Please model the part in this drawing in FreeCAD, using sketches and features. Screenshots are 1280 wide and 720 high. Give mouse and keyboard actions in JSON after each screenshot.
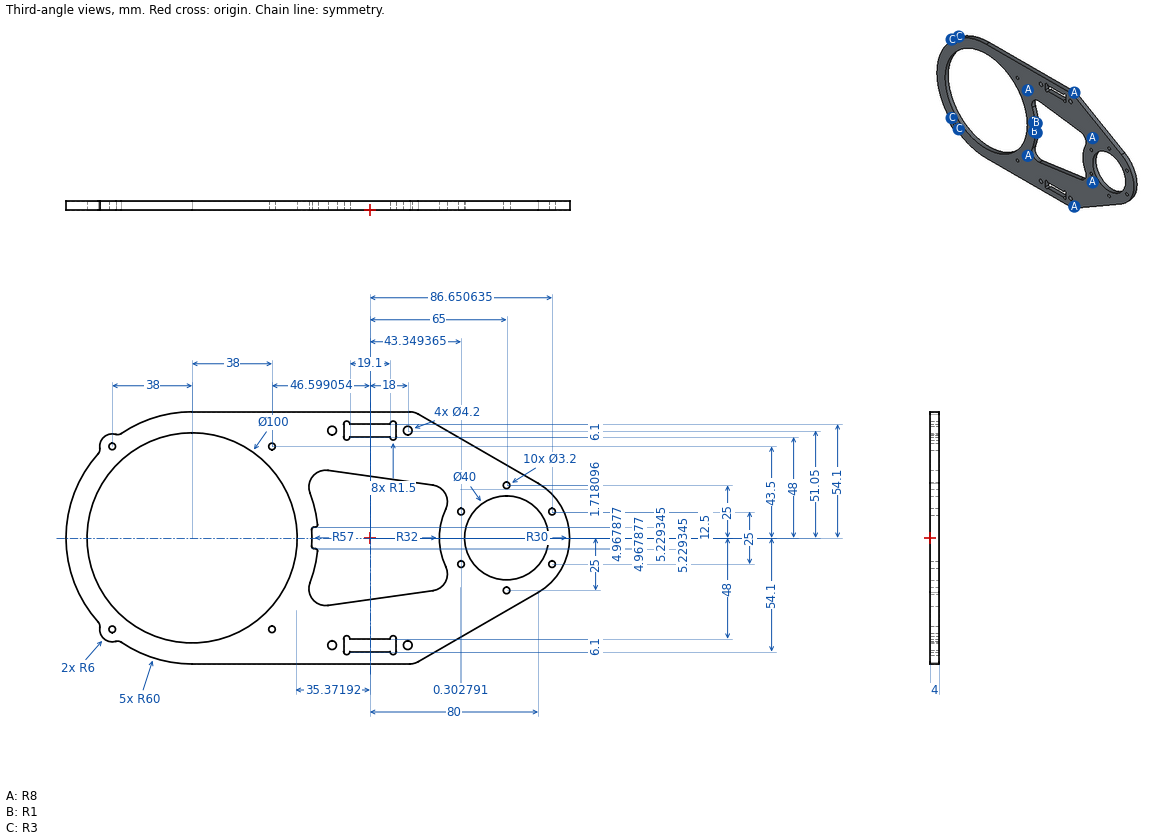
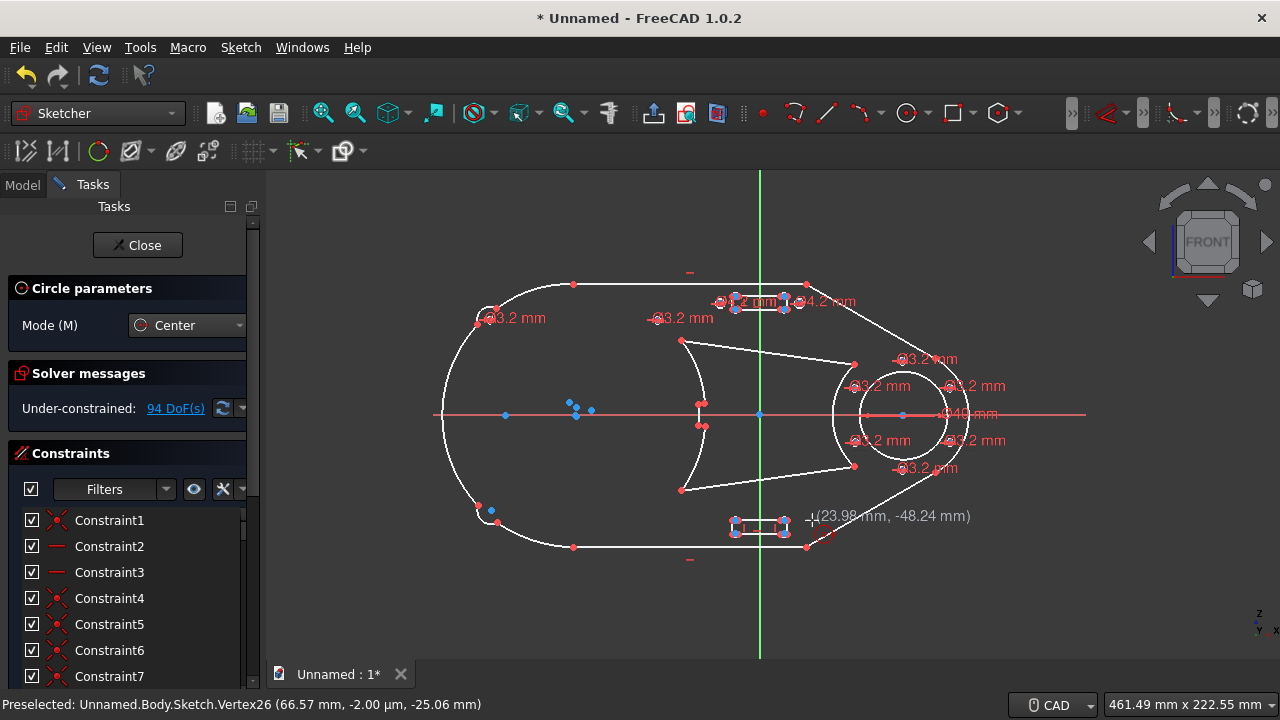
{"action": "scroll", "coordinate": [799, 527], "scroll_direction": "up", "scroll_amount": 2}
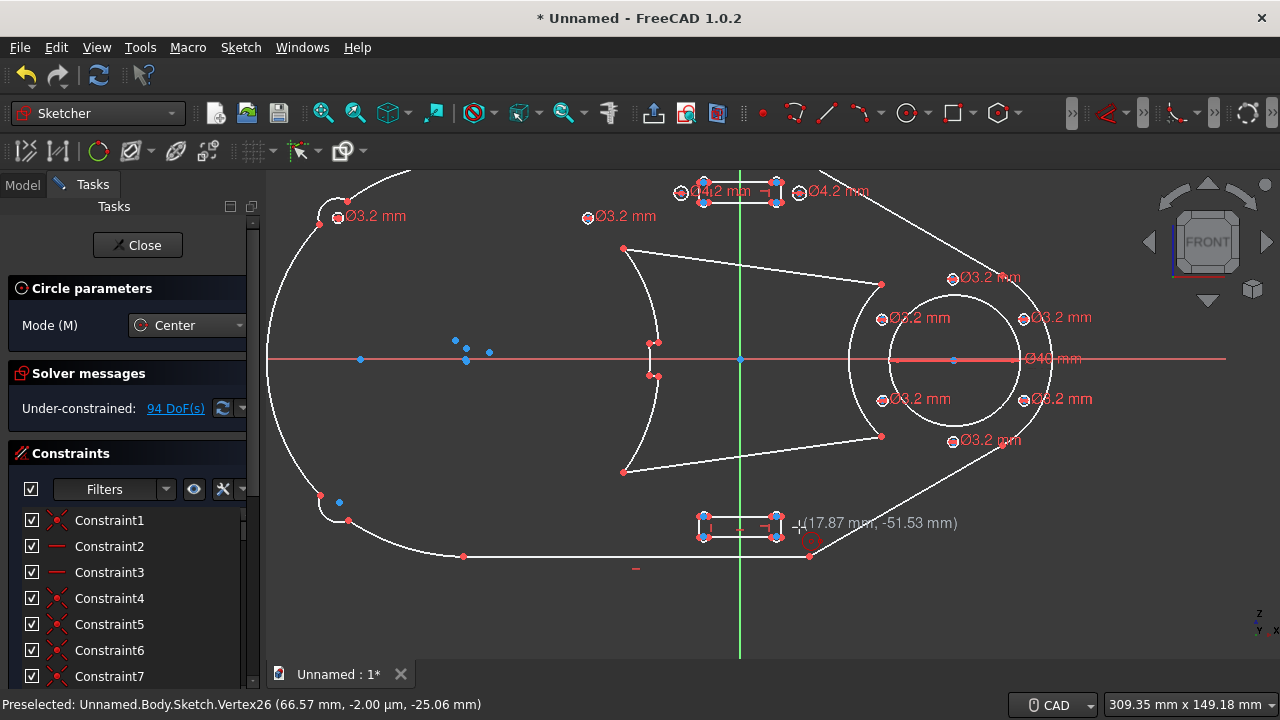
{"action": "left_click", "coordinate": [799, 527]}
{"action": "mouse_move", "coordinate": [804, 522]}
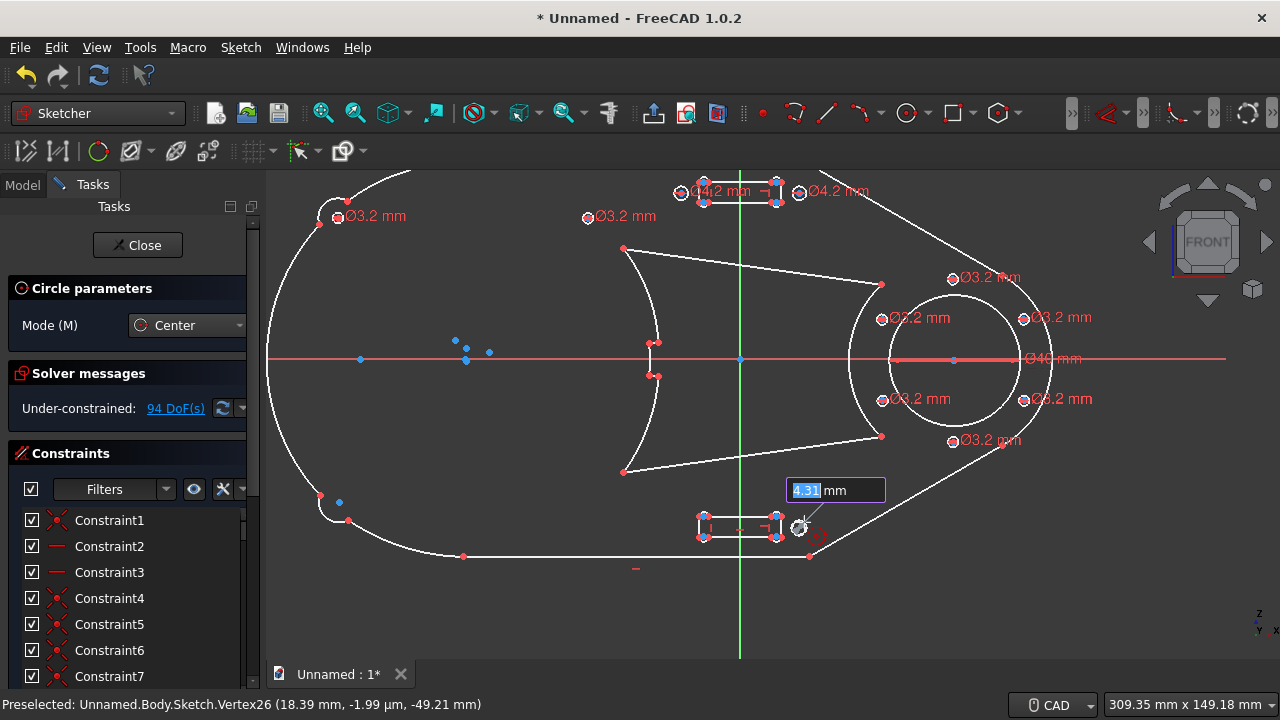
{"action": "type", "text": "4.2"}
{"action": "key", "text": "Return"}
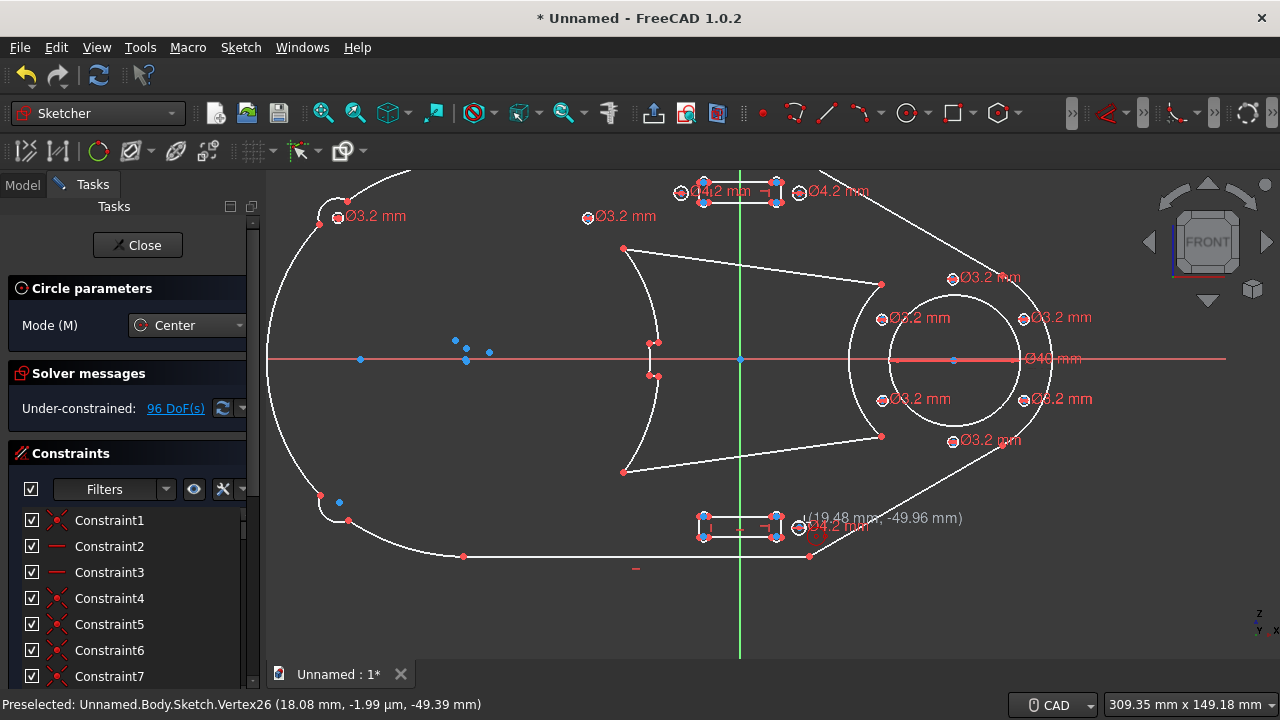
{"action": "scroll", "coordinate": [681, 527], "scroll_direction": "up", "scroll_amount": 6}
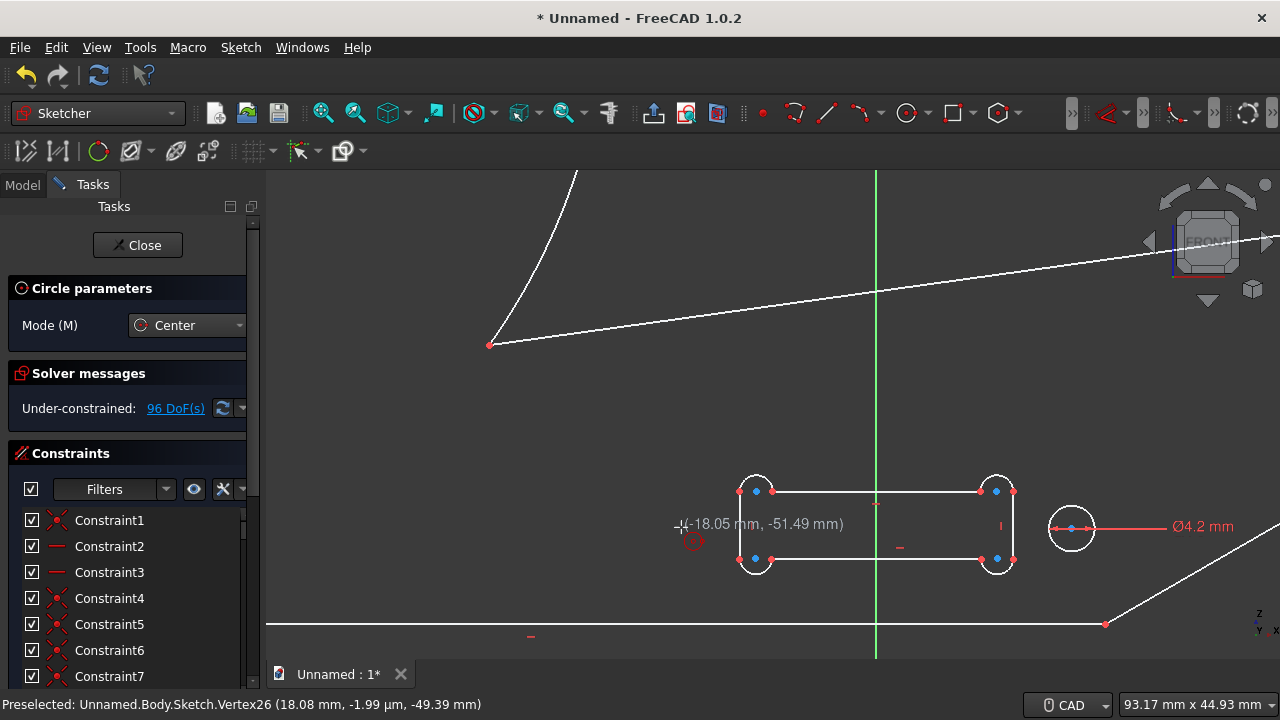
{"action": "scroll", "coordinate": [729, 527], "scroll_direction": "down", "scroll_amount": 8}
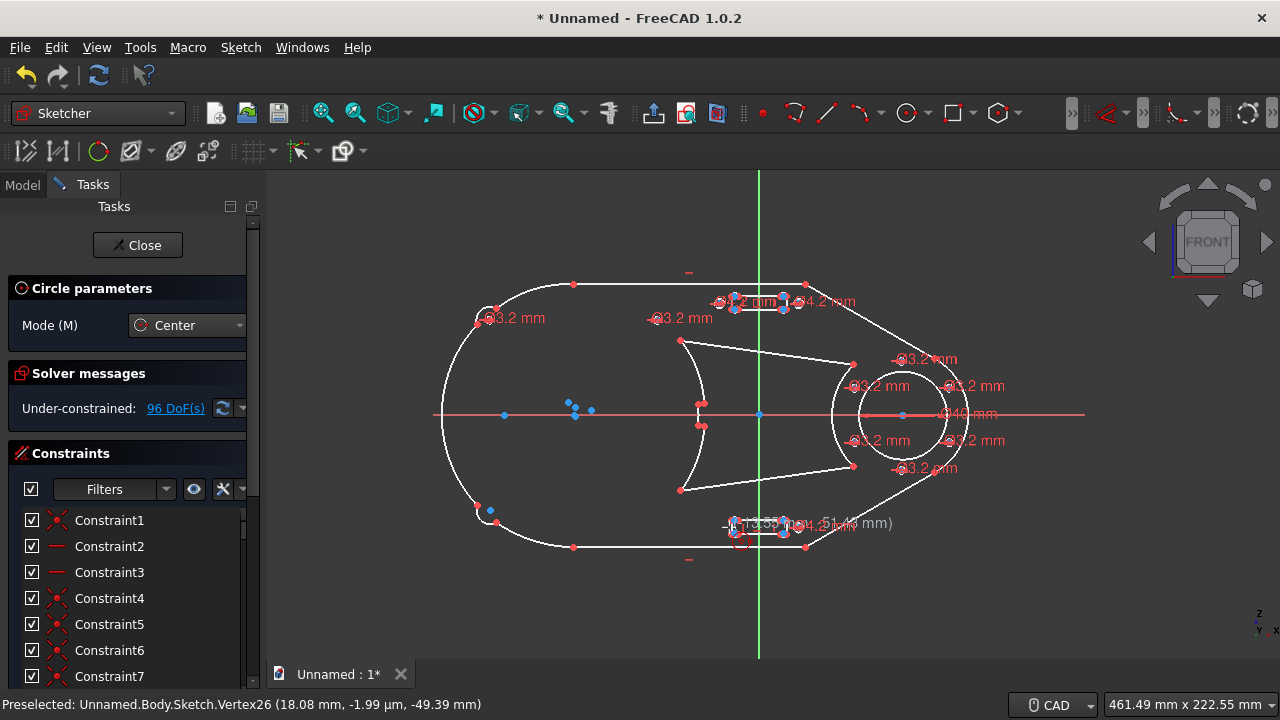
{"action": "scroll", "coordinate": [720, 527], "scroll_direction": "up", "scroll_amount": 2}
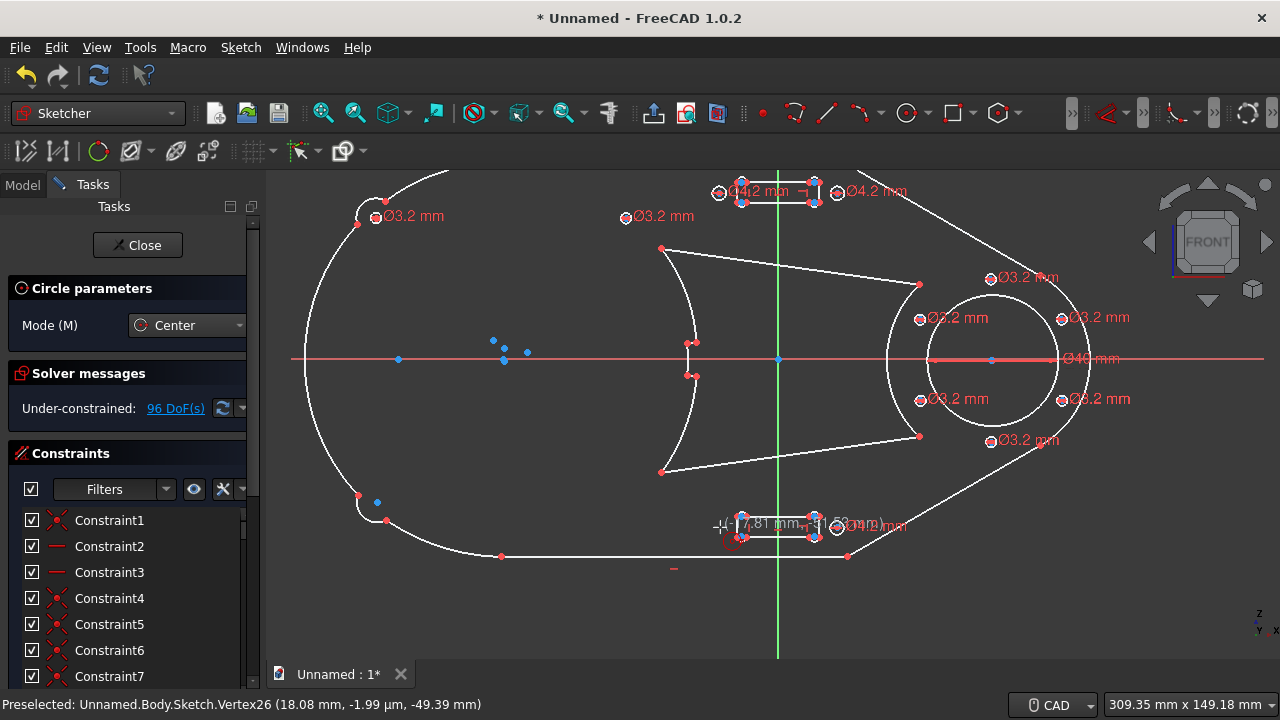
{"action": "left_click", "coordinate": [719, 527]}
{"action": "mouse_move", "coordinate": [714, 522]}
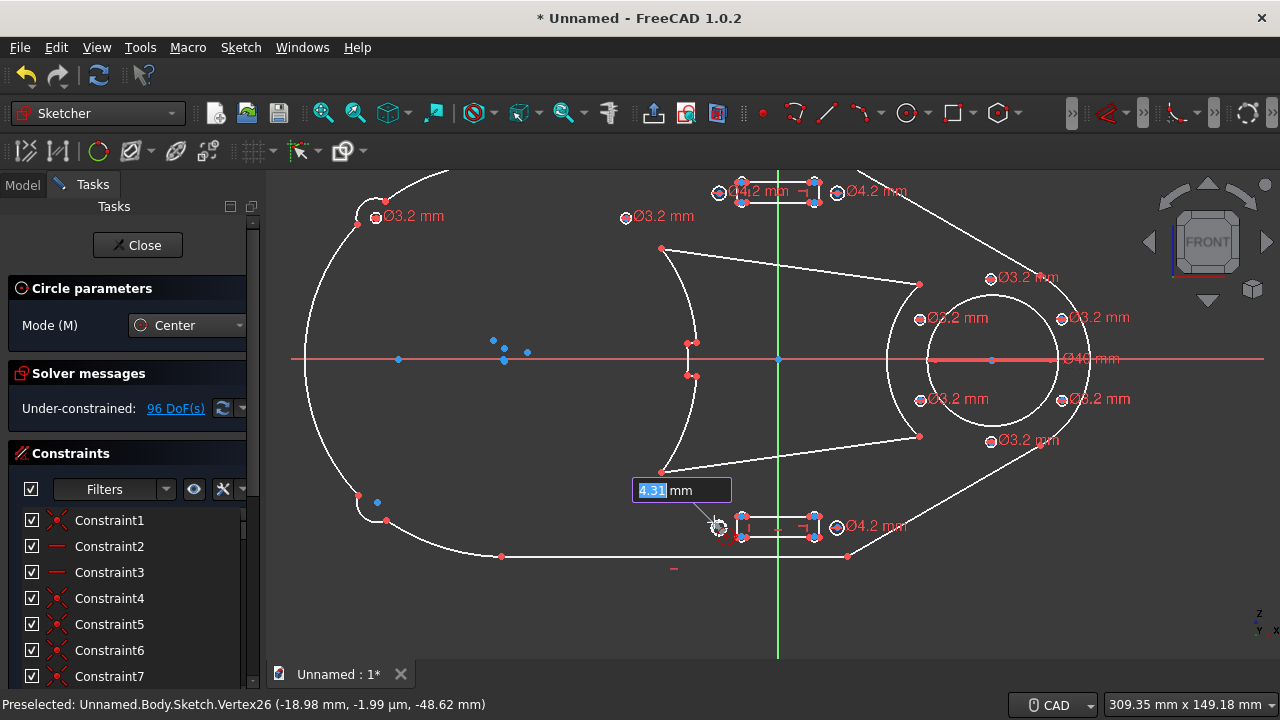
{"action": "type", "text": "4.2"}
{"action": "key", "text": "Return"}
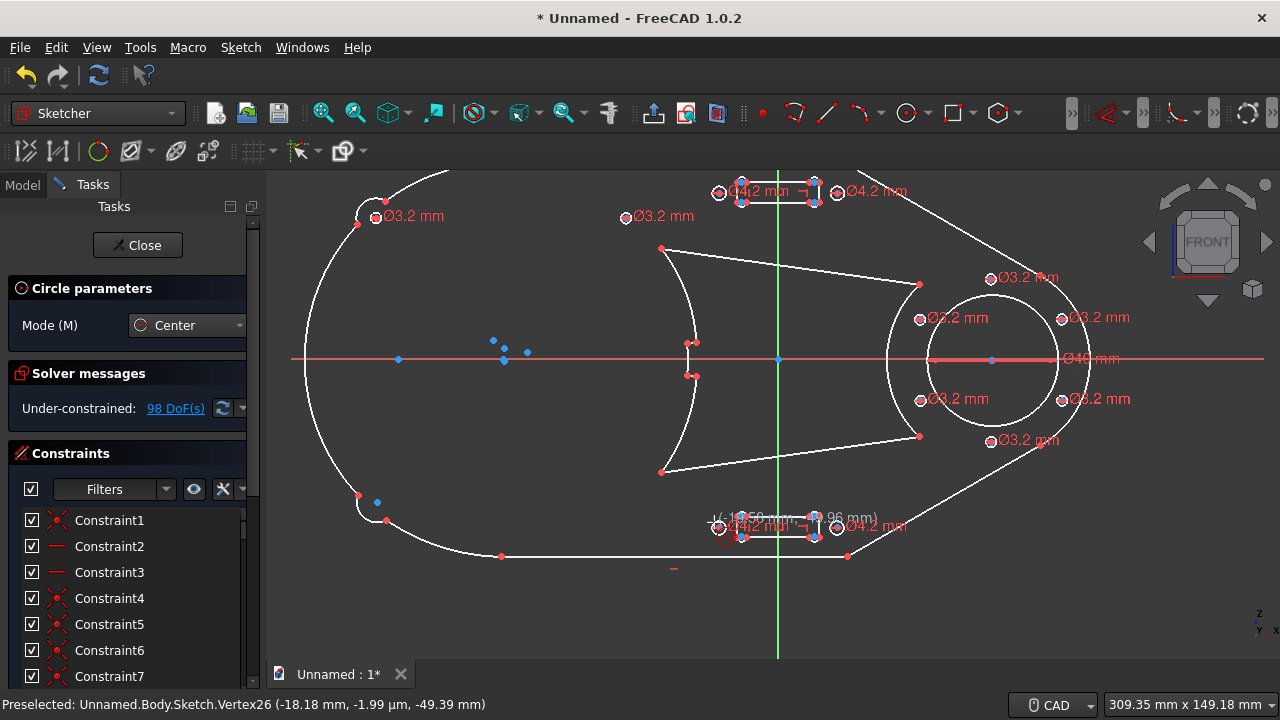
{"action": "left_click", "coordinate": [501, 359]}
{"action": "mouse_move", "coordinate": [617, 243]}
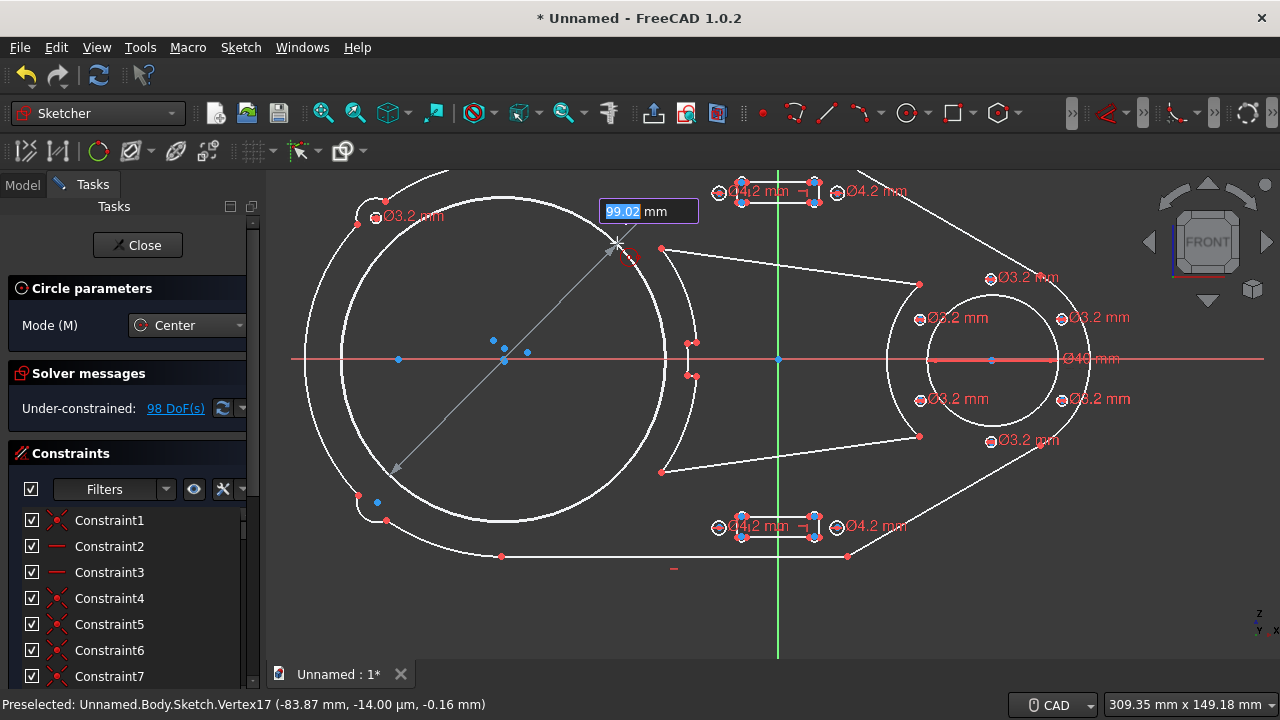
{"action": "type", "text": "100"}
{"action": "key", "text": "Return"}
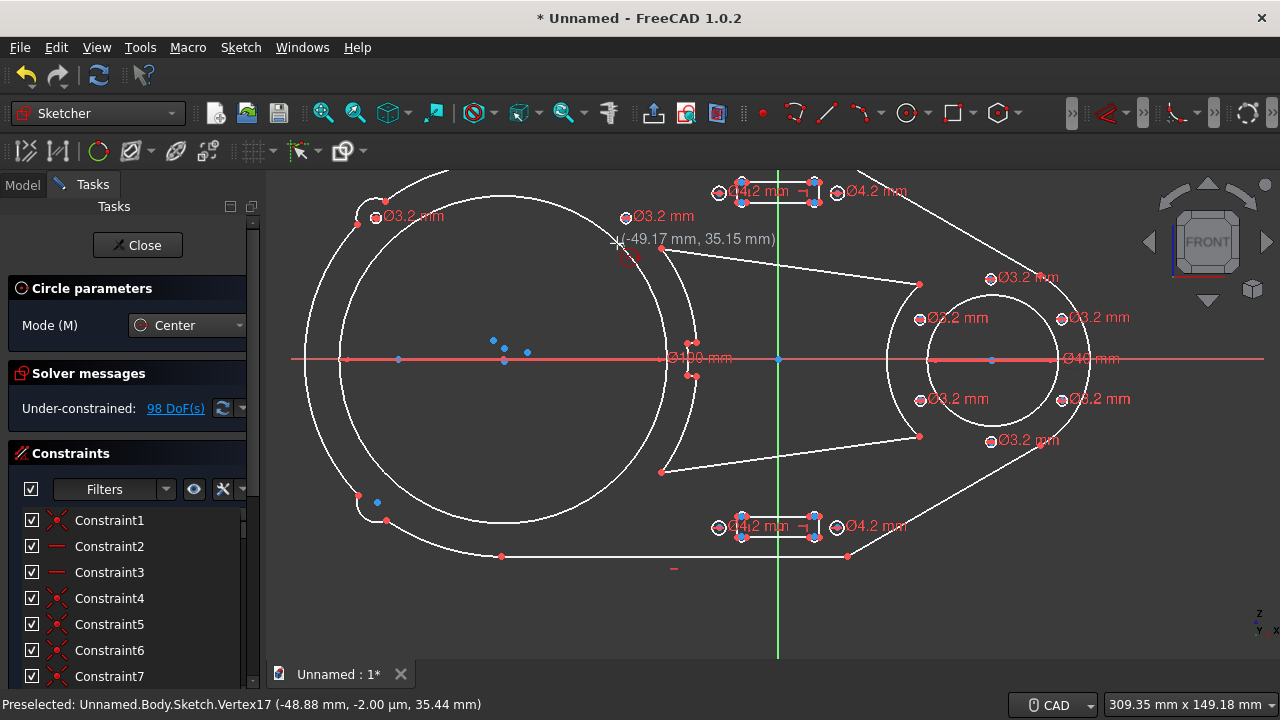
{"action": "scroll", "coordinate": [625, 502], "scroll_direction": "up", "scroll_amount": 8}